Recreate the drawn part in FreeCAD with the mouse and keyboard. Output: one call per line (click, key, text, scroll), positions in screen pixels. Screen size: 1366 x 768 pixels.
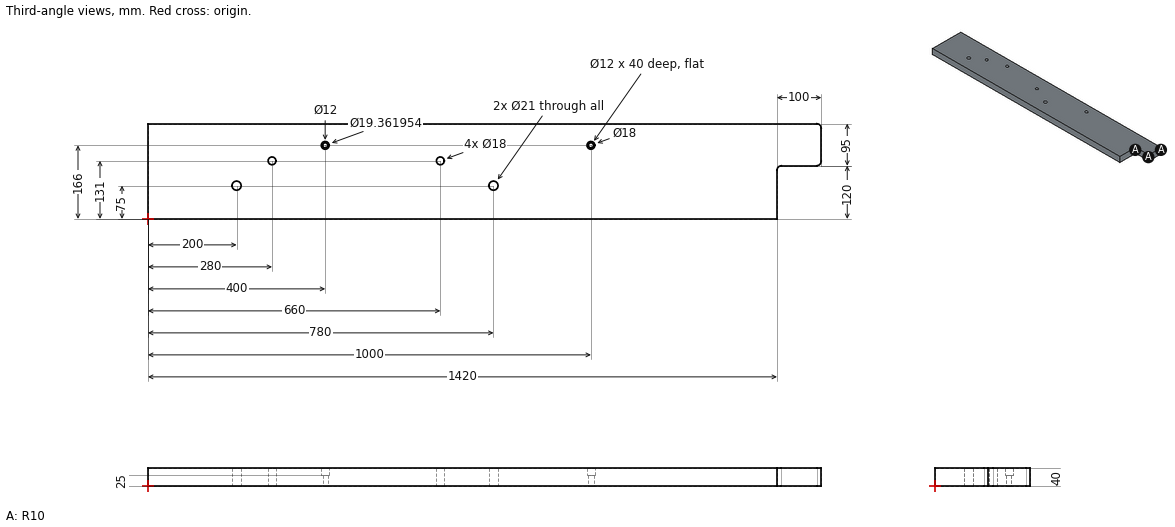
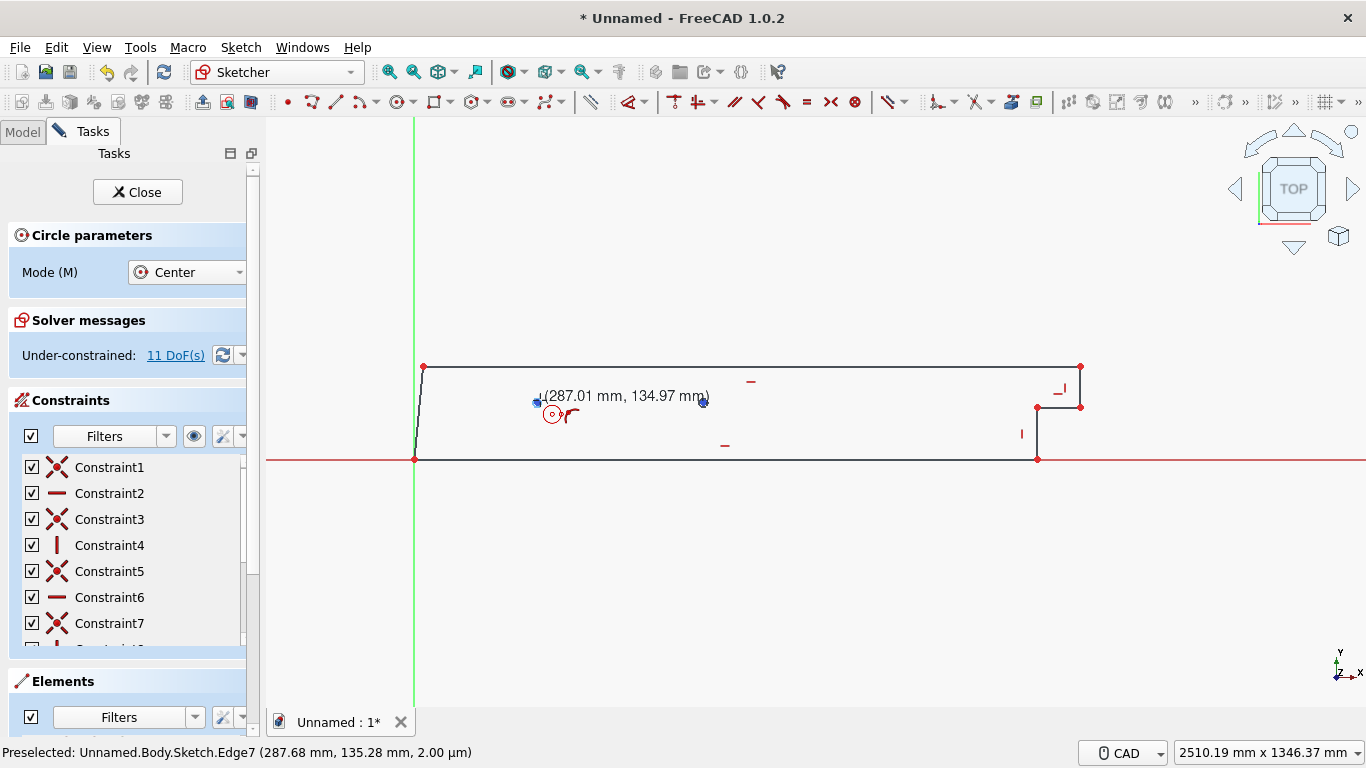
scroll(853, 387, up, 9)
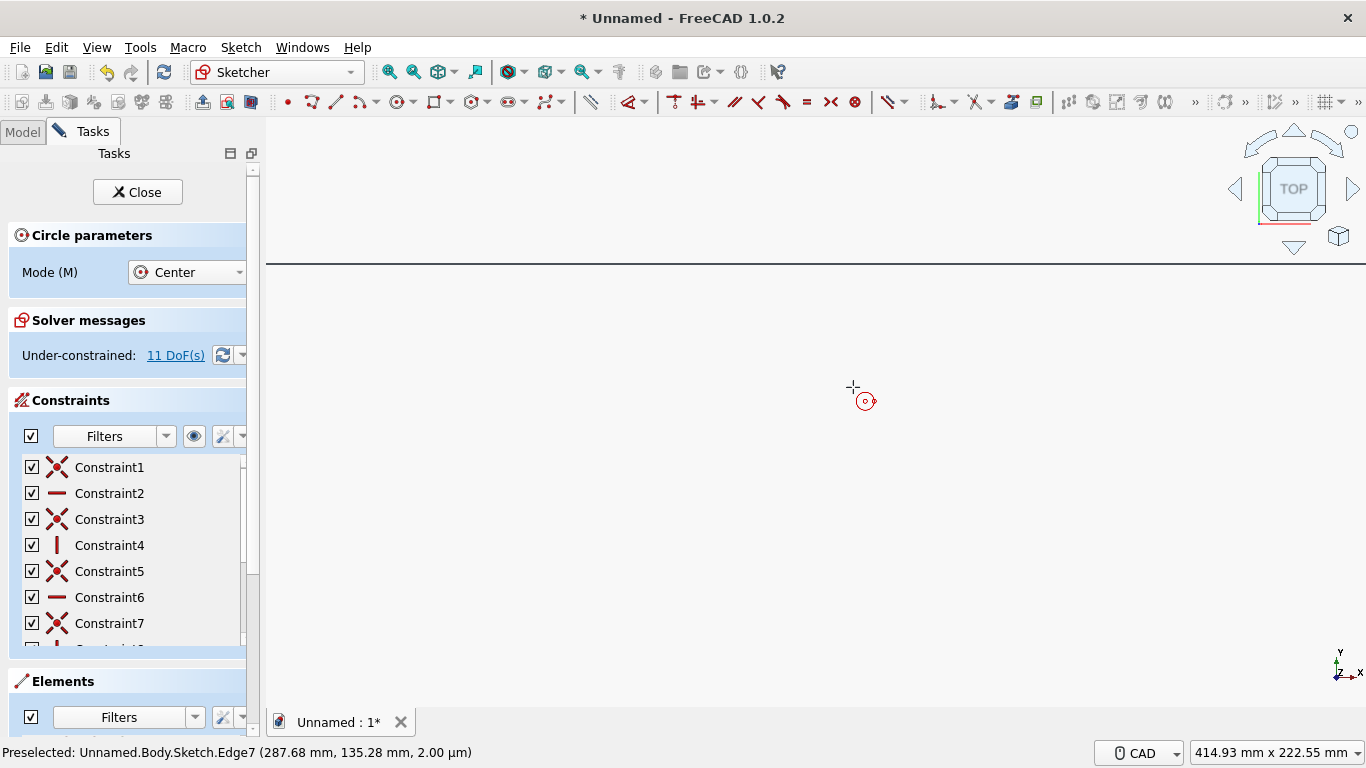
scroll(854, 387, down, 9)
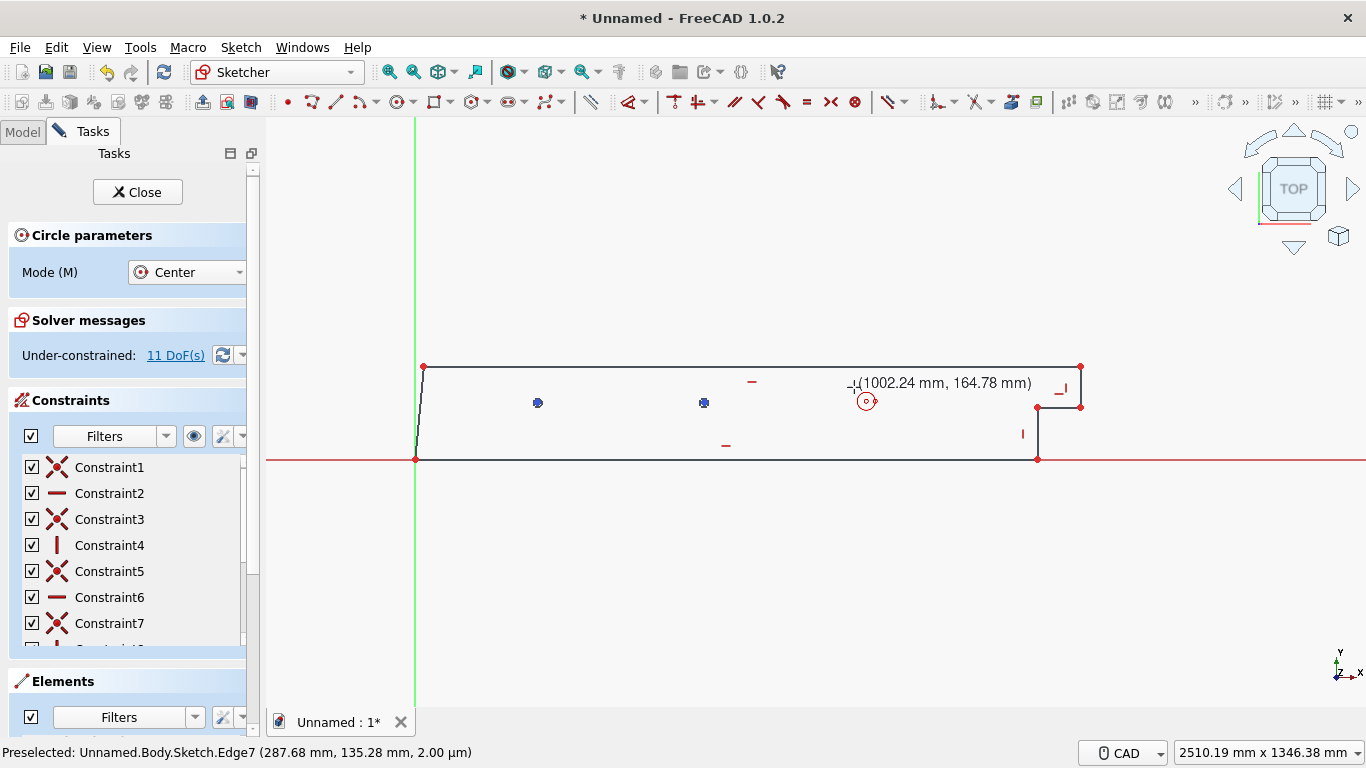
click(853, 387)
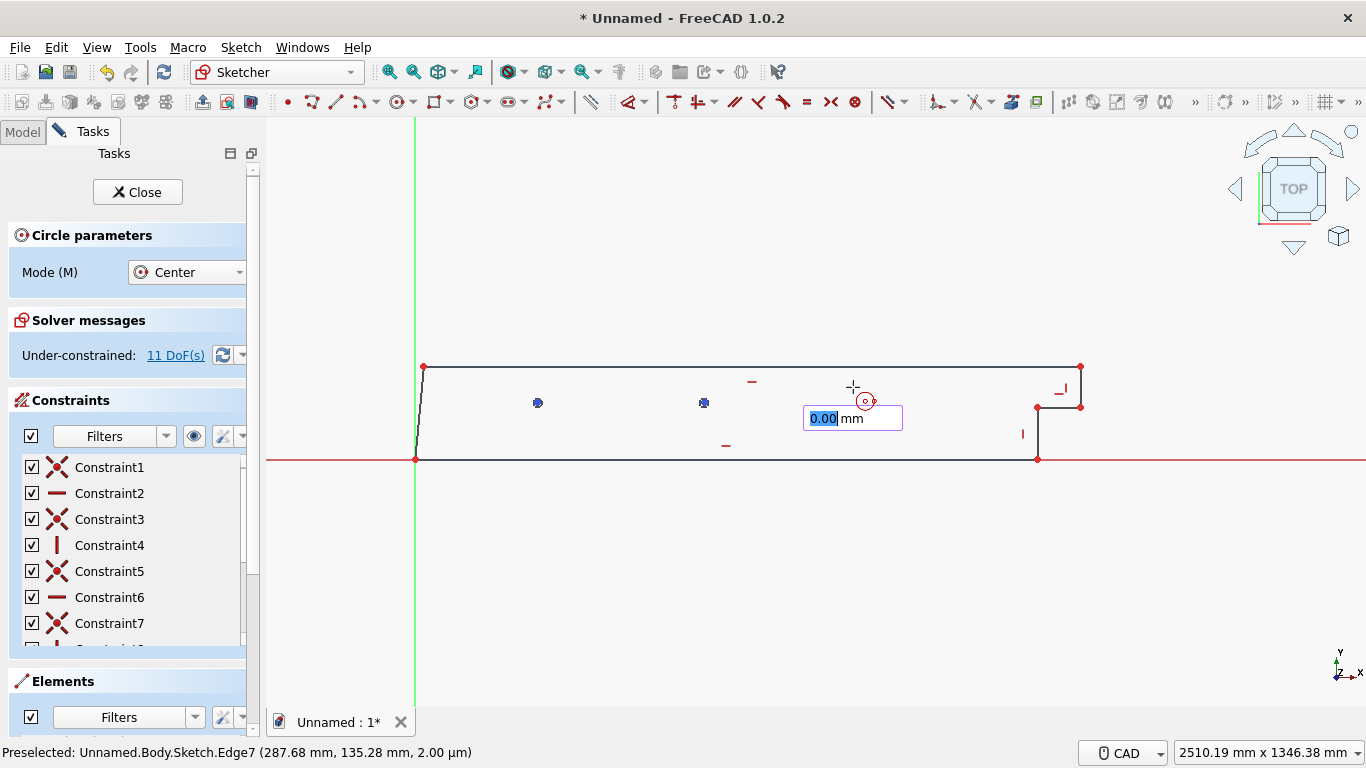
scroll(856, 384, up, 7)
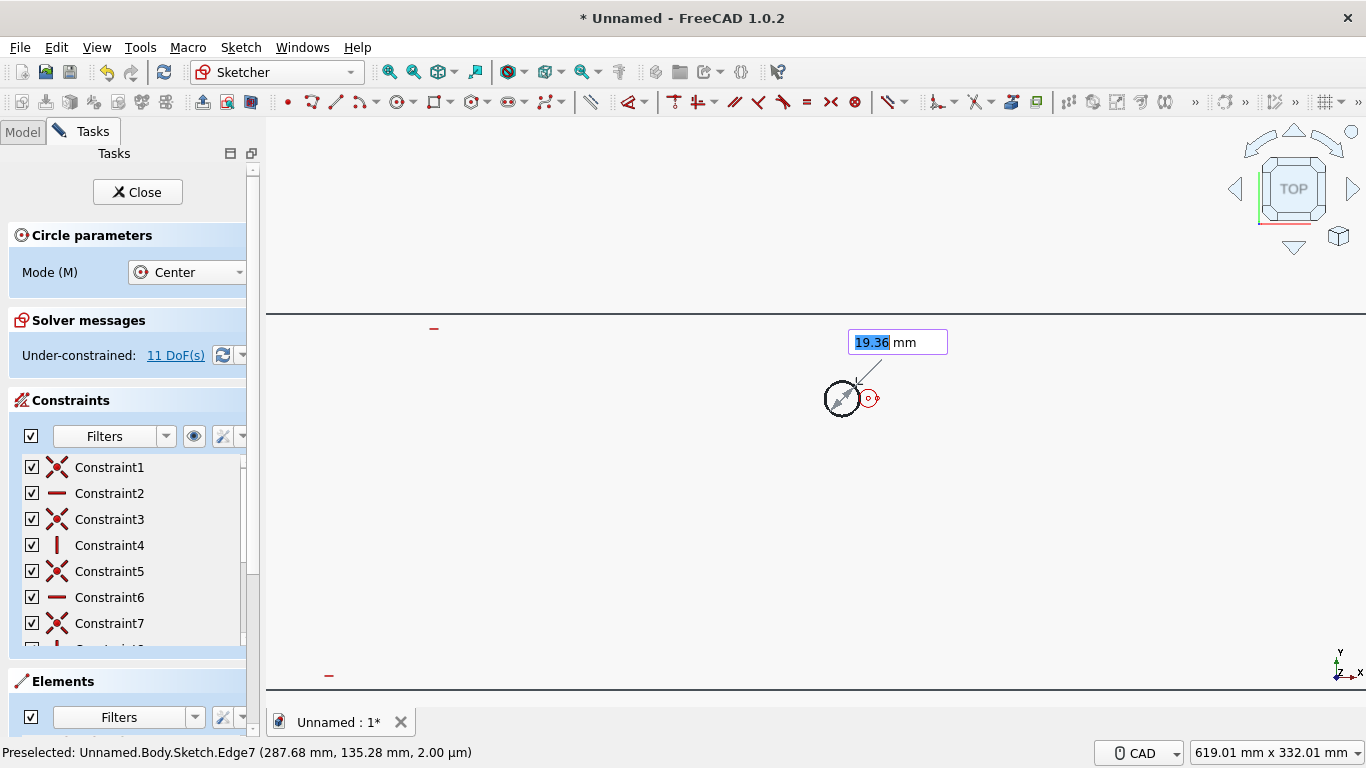
click(855, 384)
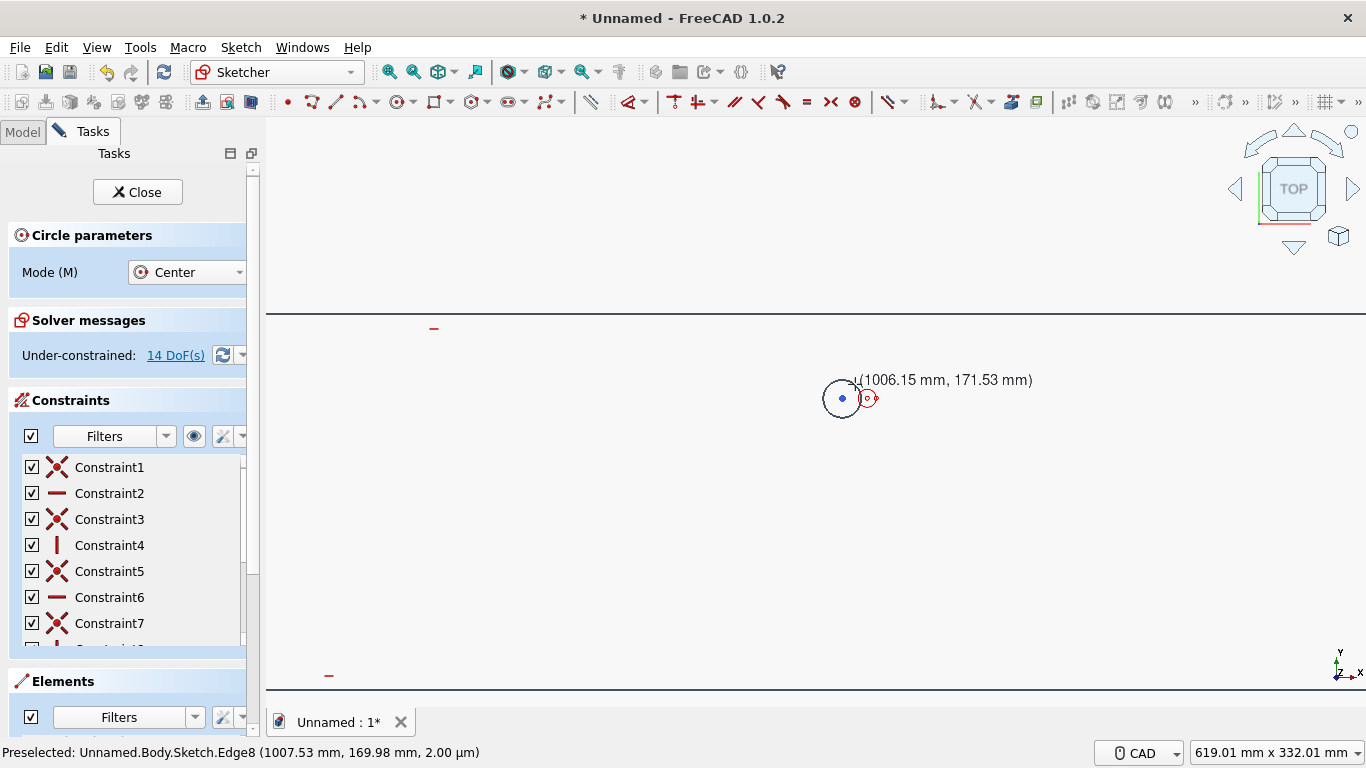
scroll(855, 384, down, 7)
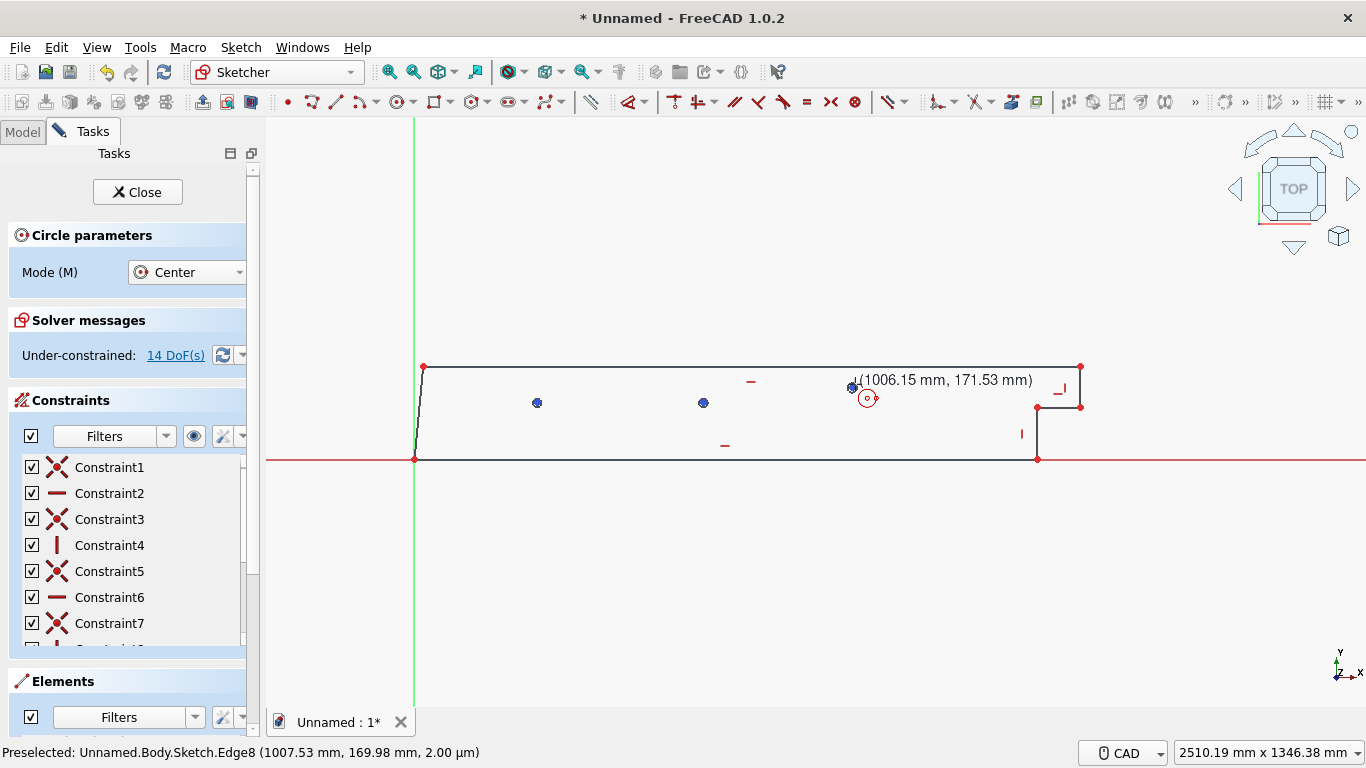
scroll(590, 387, up, 9)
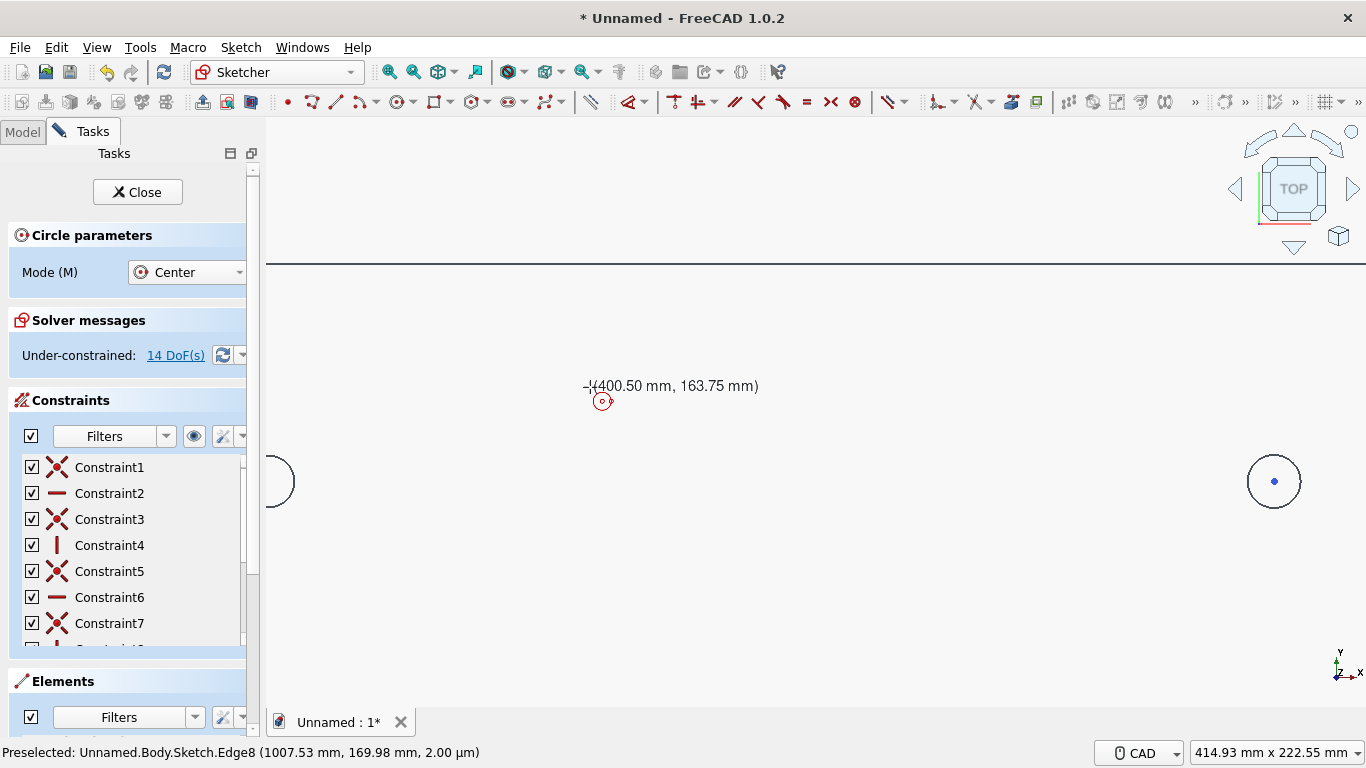
scroll(590, 387, down, 9)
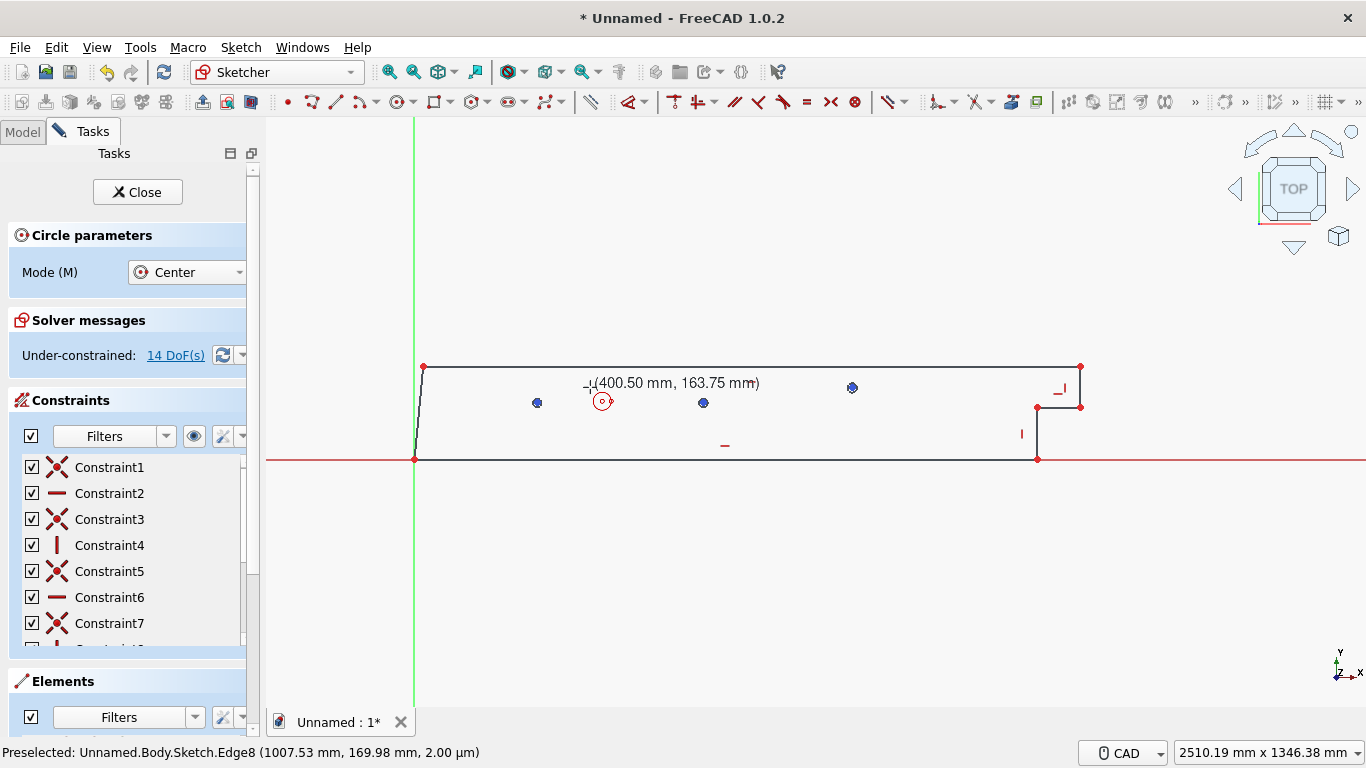
click(590, 387)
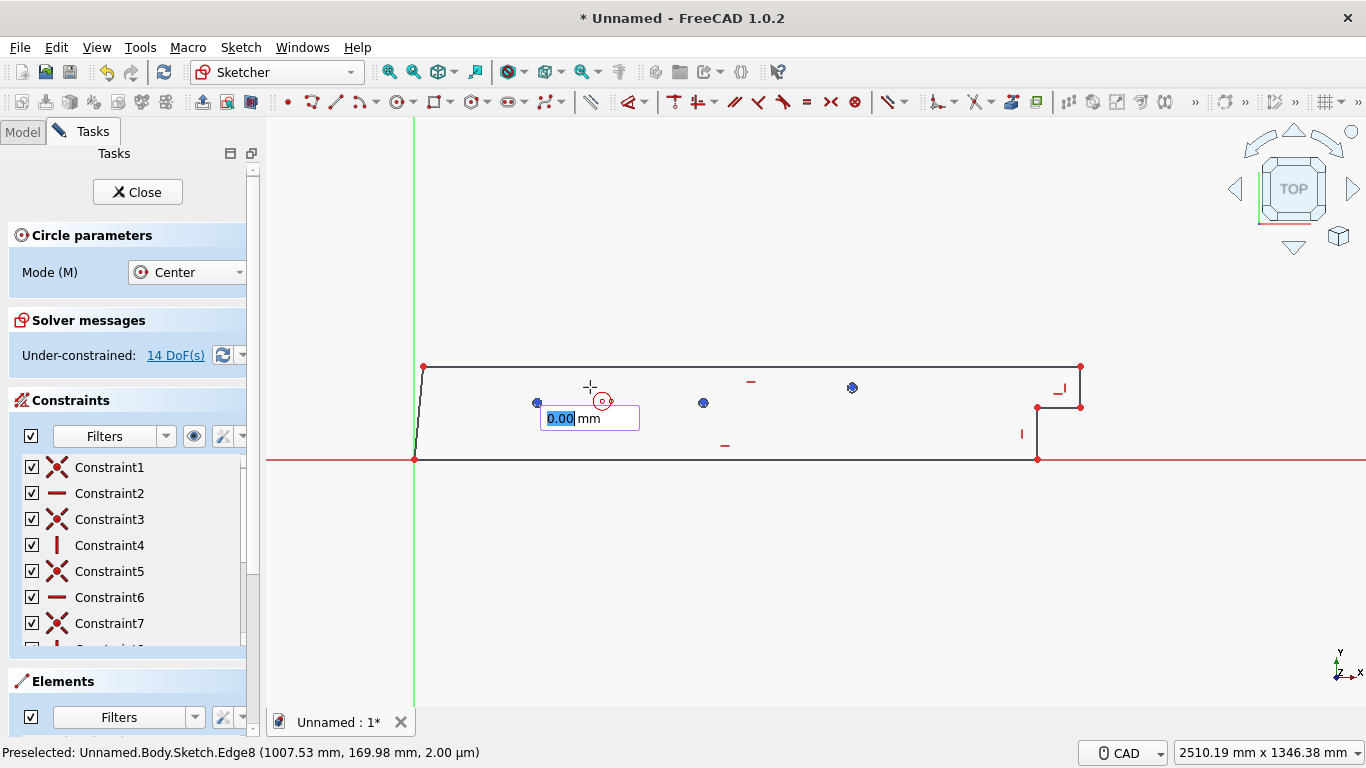
scroll(593, 384, up, 7)